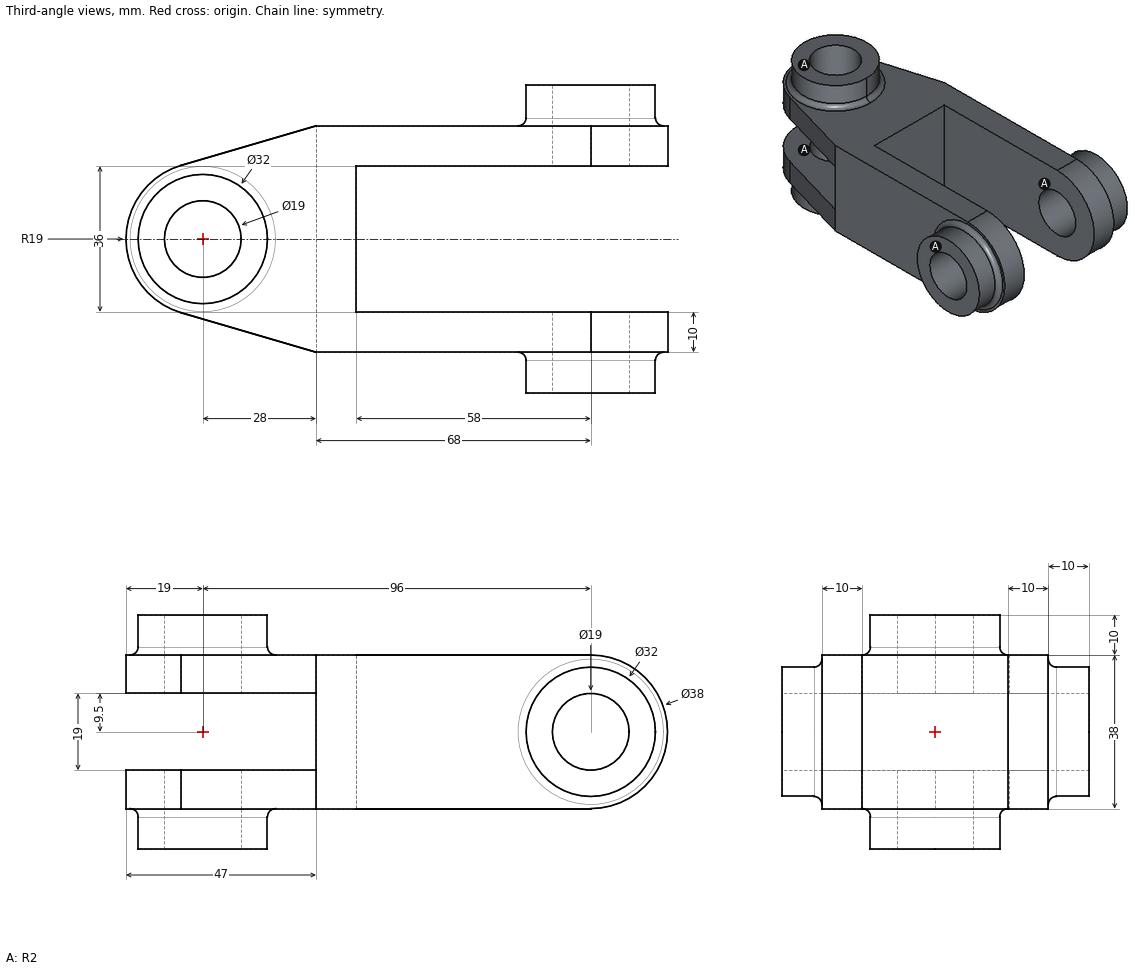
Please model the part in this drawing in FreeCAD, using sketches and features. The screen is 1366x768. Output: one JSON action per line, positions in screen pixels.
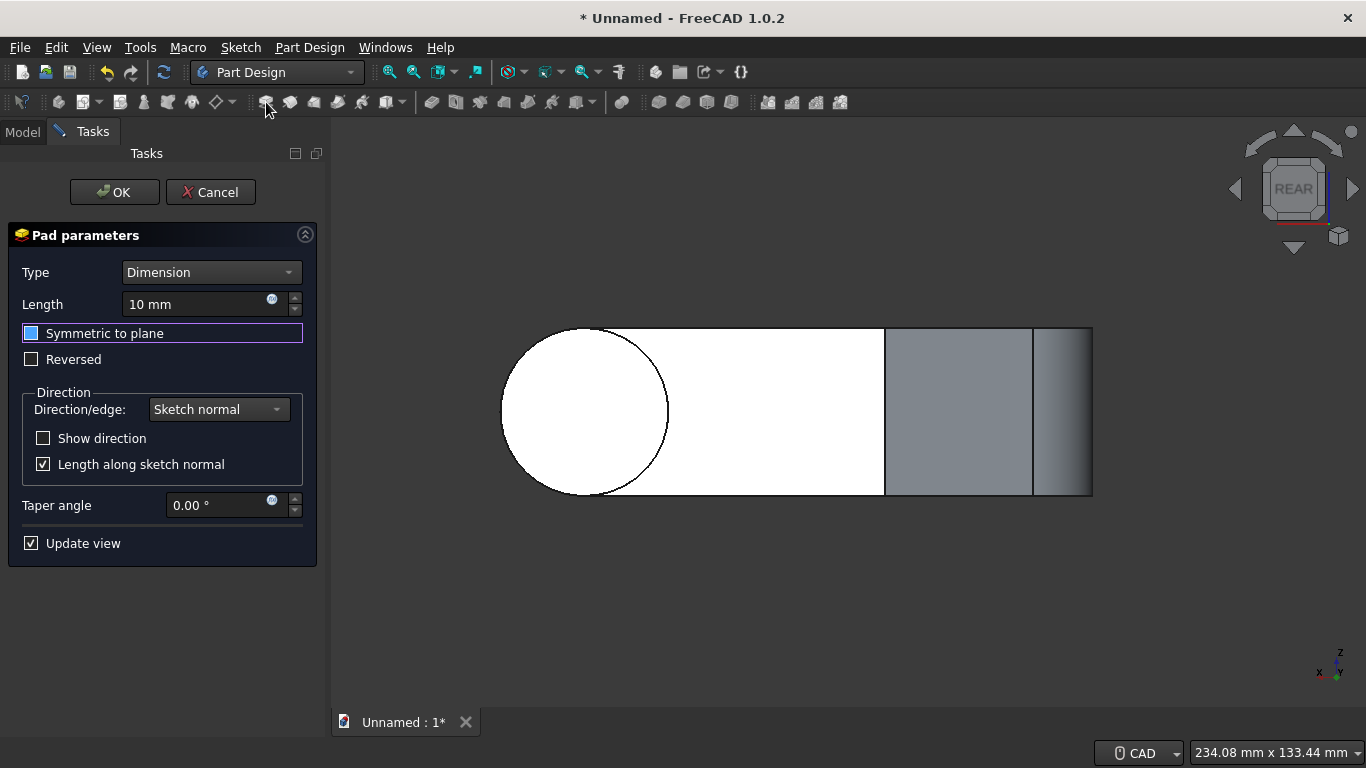
{"action": "left_click", "coordinate": [30, 359]}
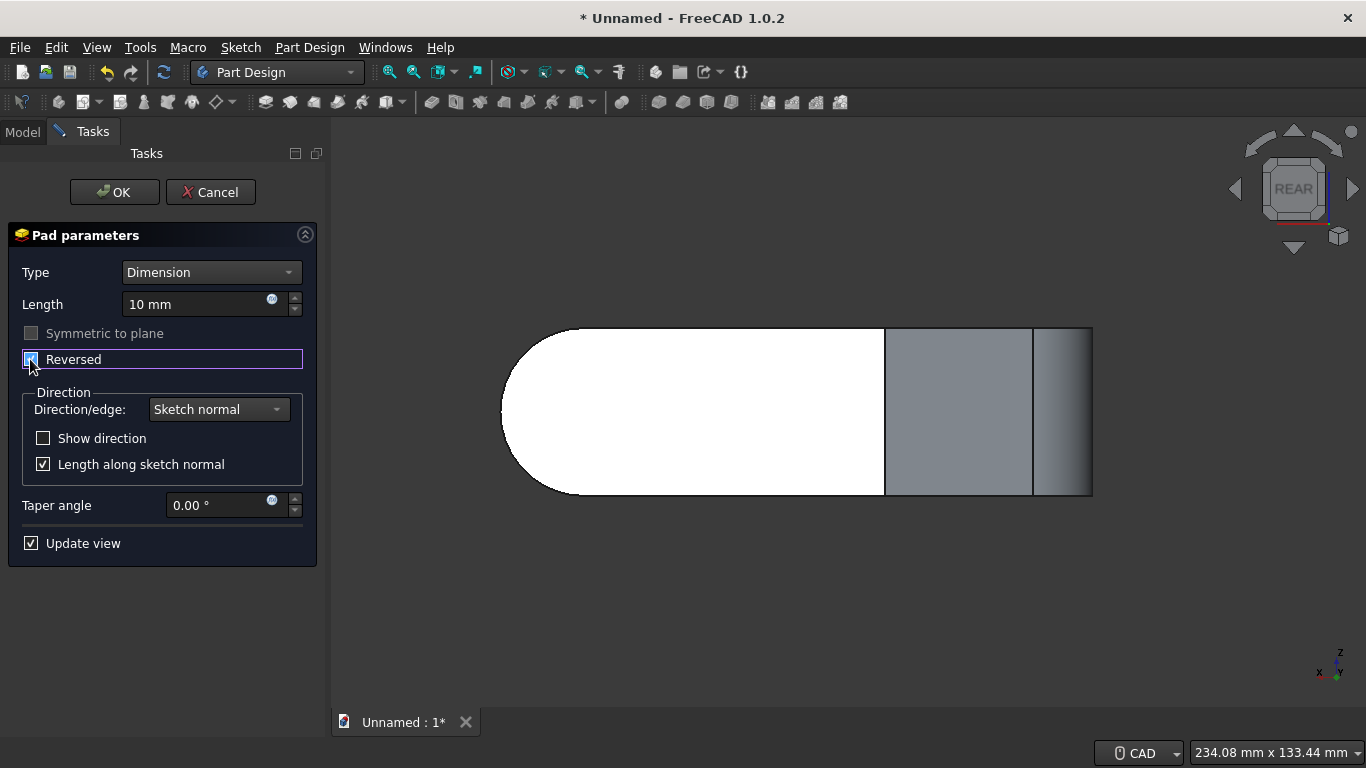
{"action": "left_click", "coordinate": [115, 192]}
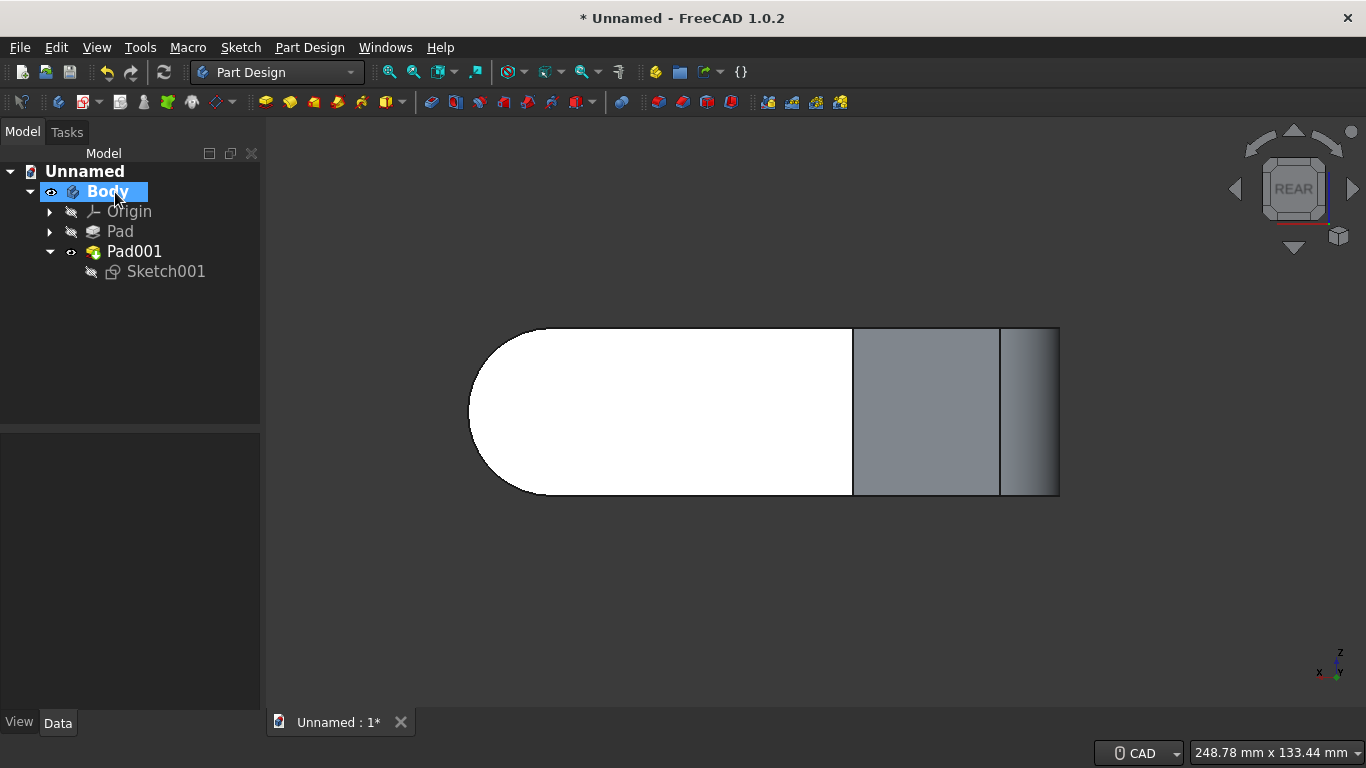
{"action": "left_click", "coordinate": [50, 212]}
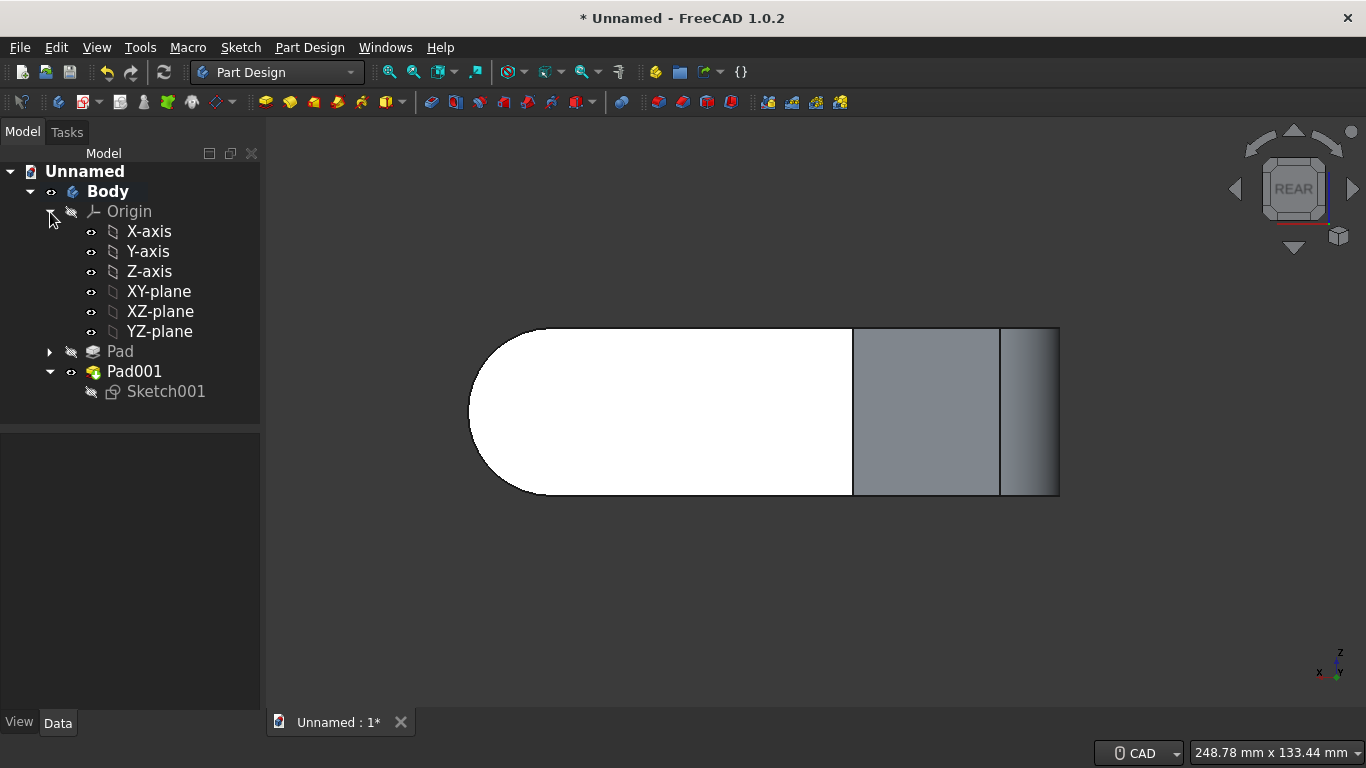
{"action": "left_click", "coordinate": [136, 312]}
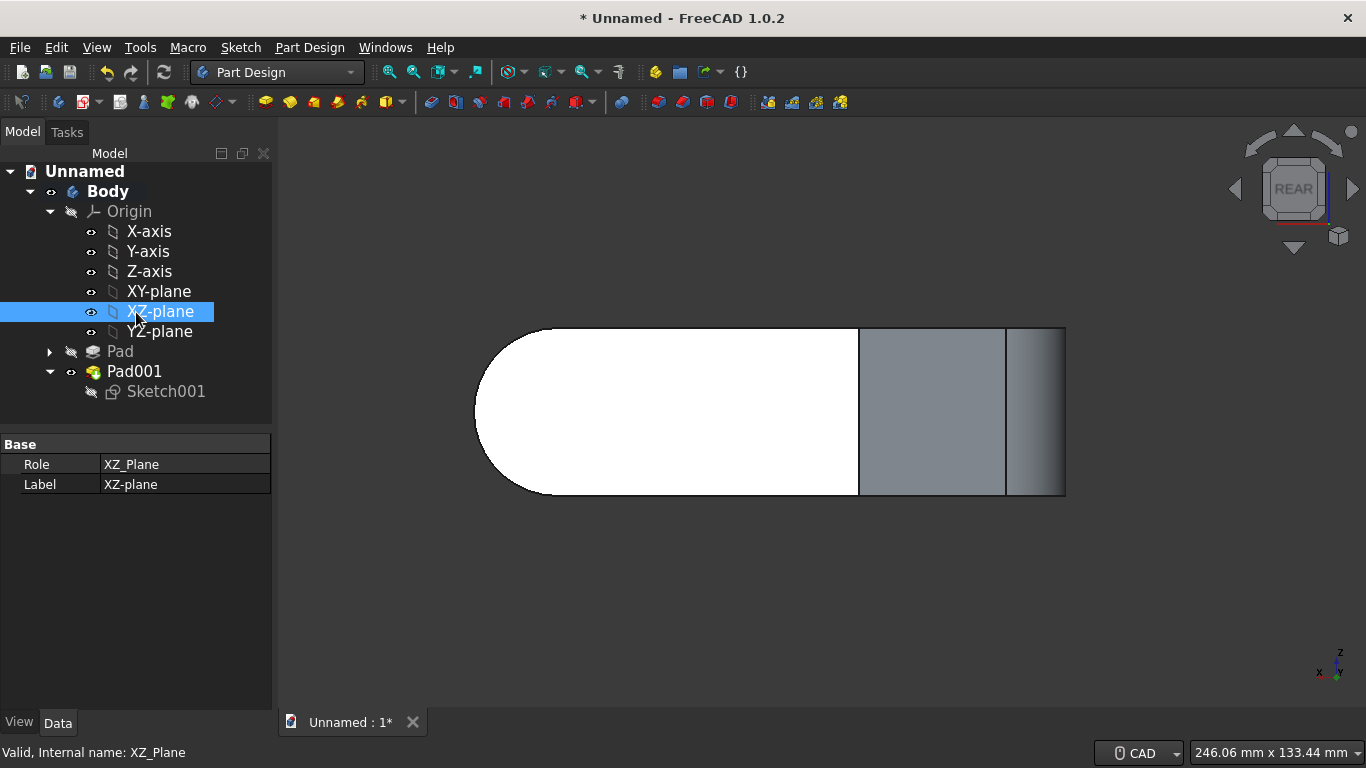
{"action": "left_click", "coordinate": [216, 102]}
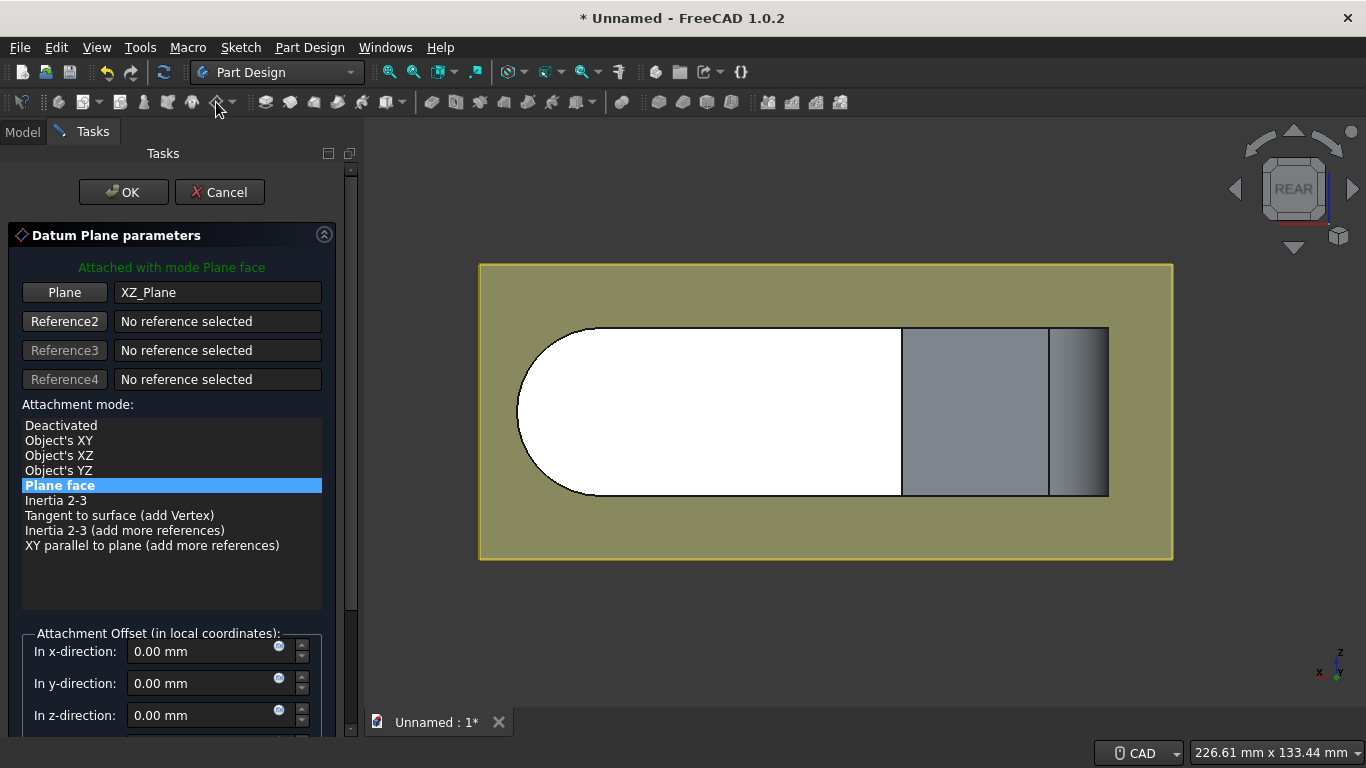
{"action": "triple_click", "coordinate": [210, 715]}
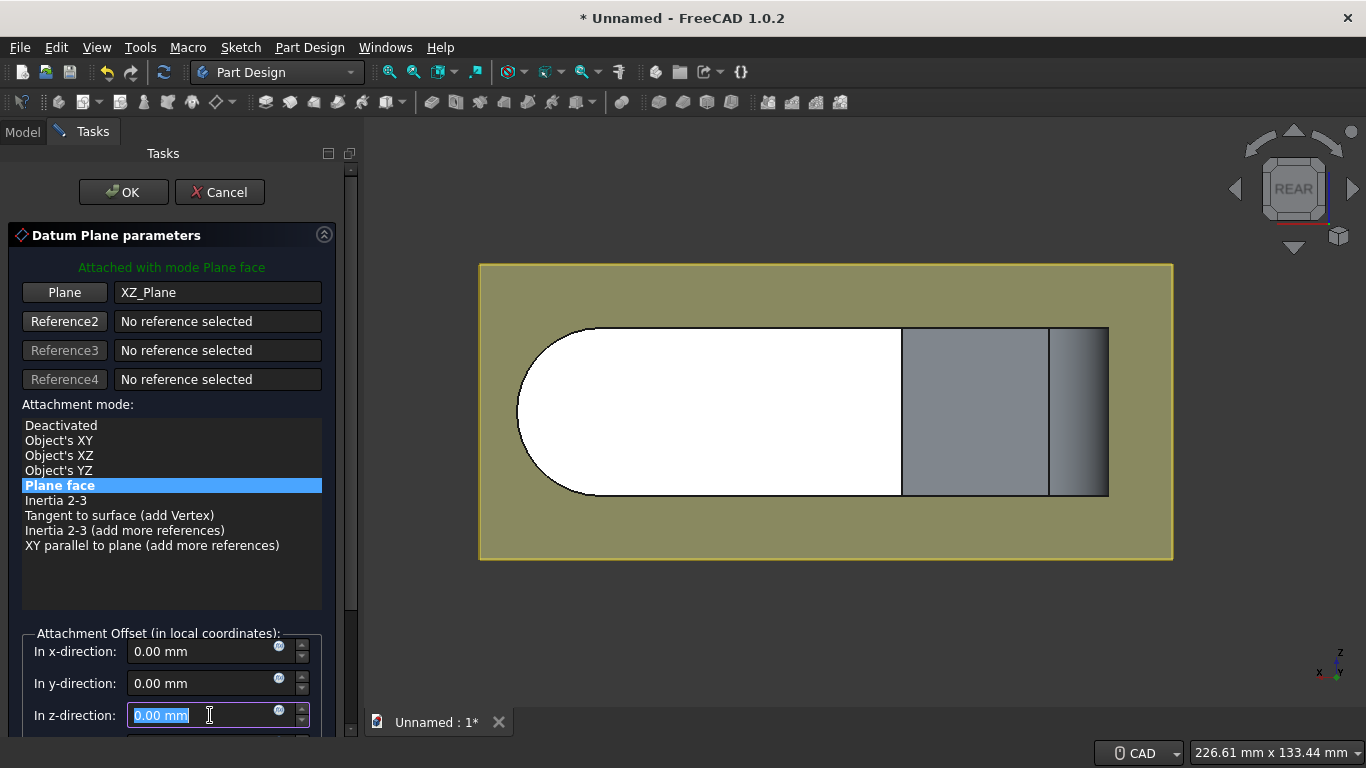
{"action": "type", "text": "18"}
{"action": "key", "text": "Tab"}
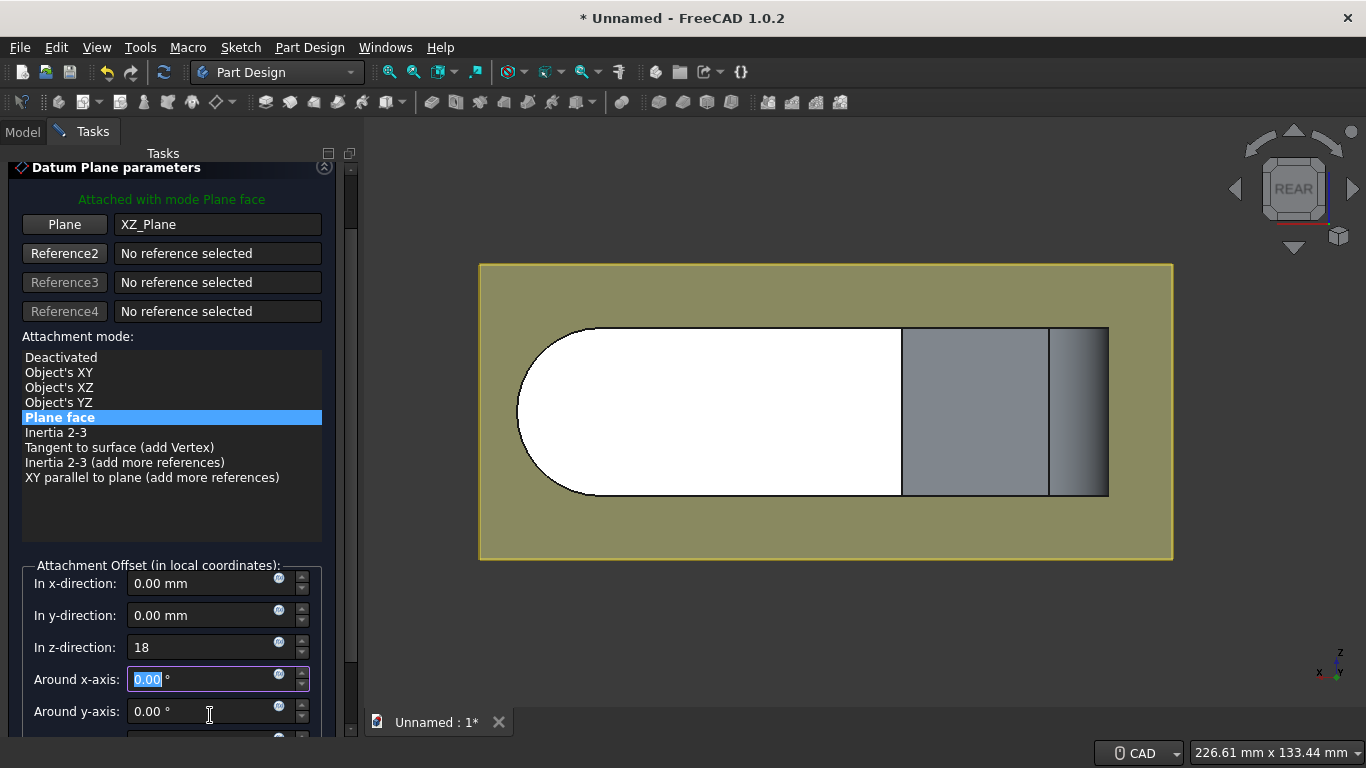
{"action": "scroll", "coordinate": [351, 450], "scroll_direction": "up", "scroll_amount": 2}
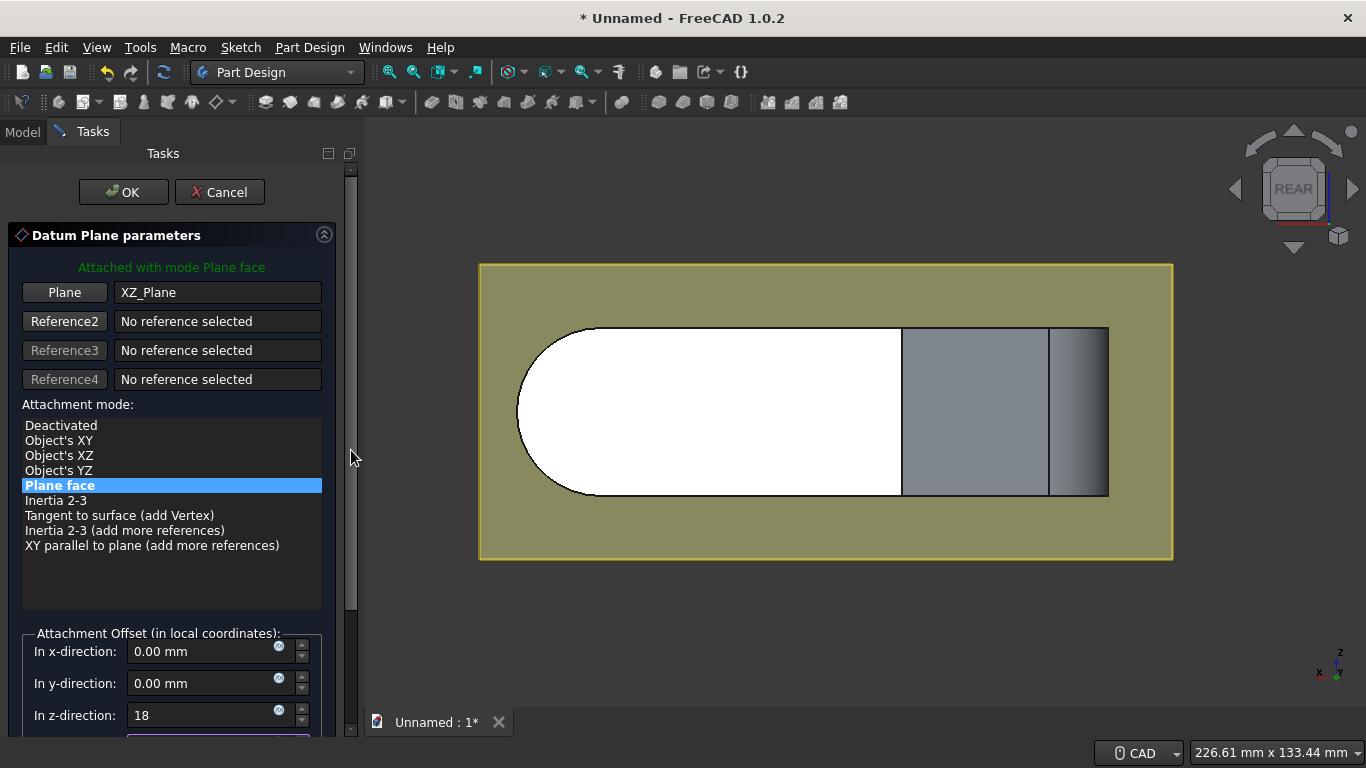
{"action": "left_click", "coordinate": [124, 192]}